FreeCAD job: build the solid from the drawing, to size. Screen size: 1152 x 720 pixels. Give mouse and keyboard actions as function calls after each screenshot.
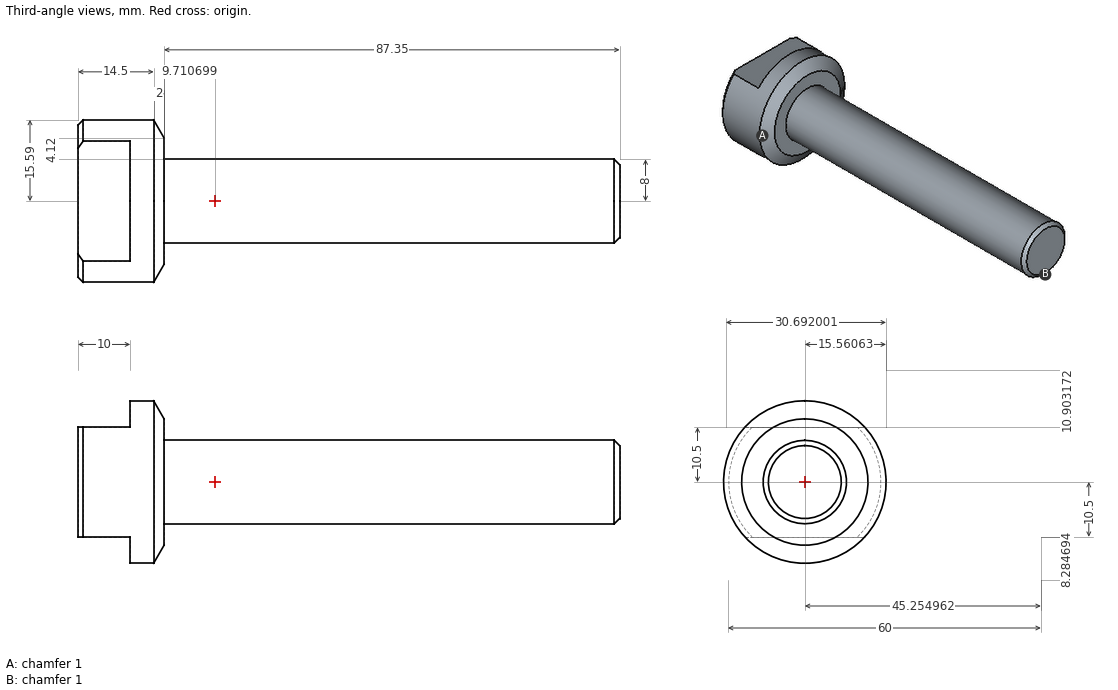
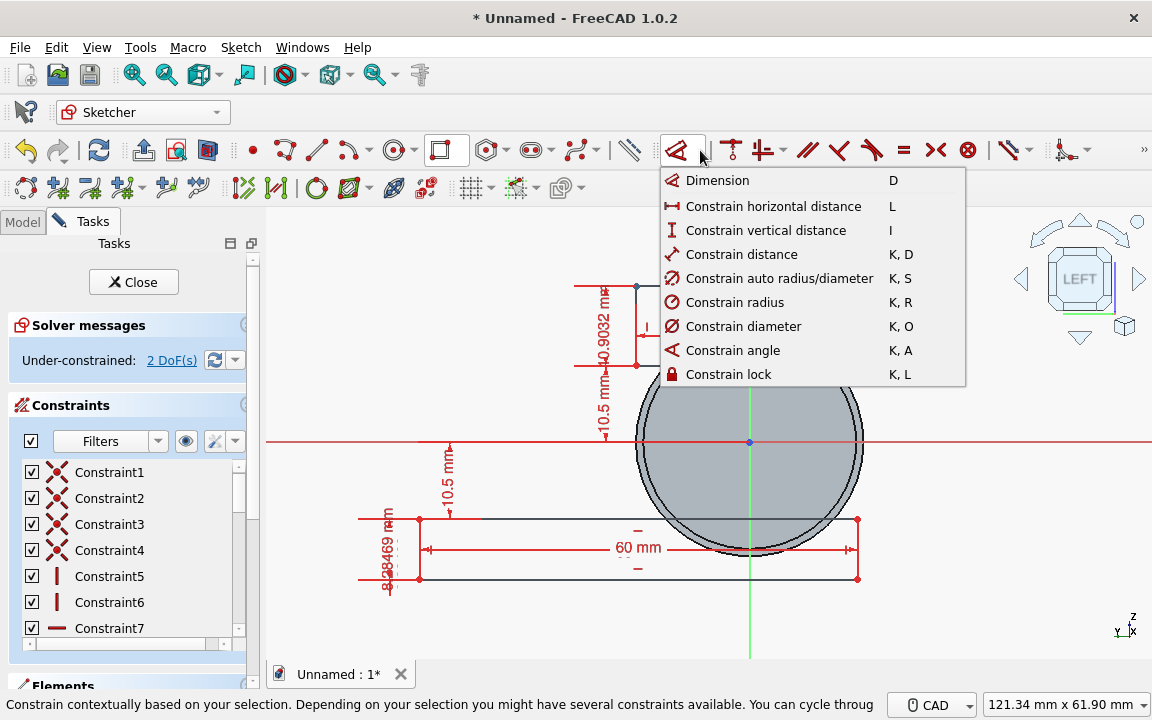
click(813, 206)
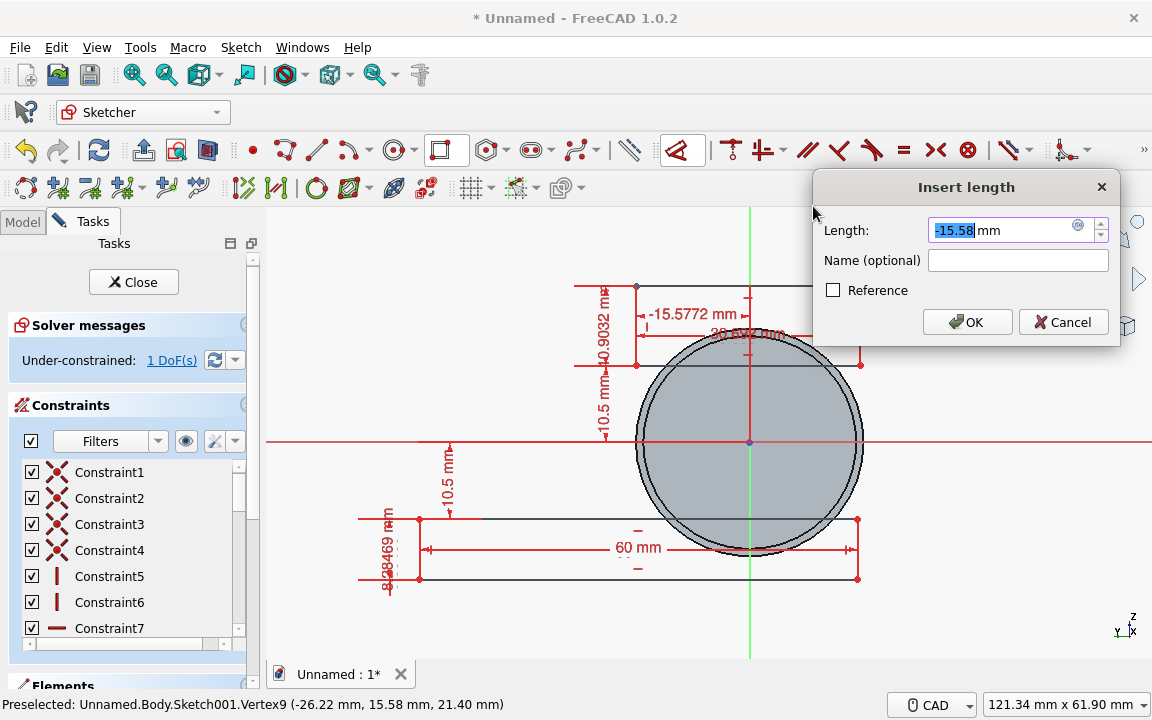
text(-15.56063)
key(Return)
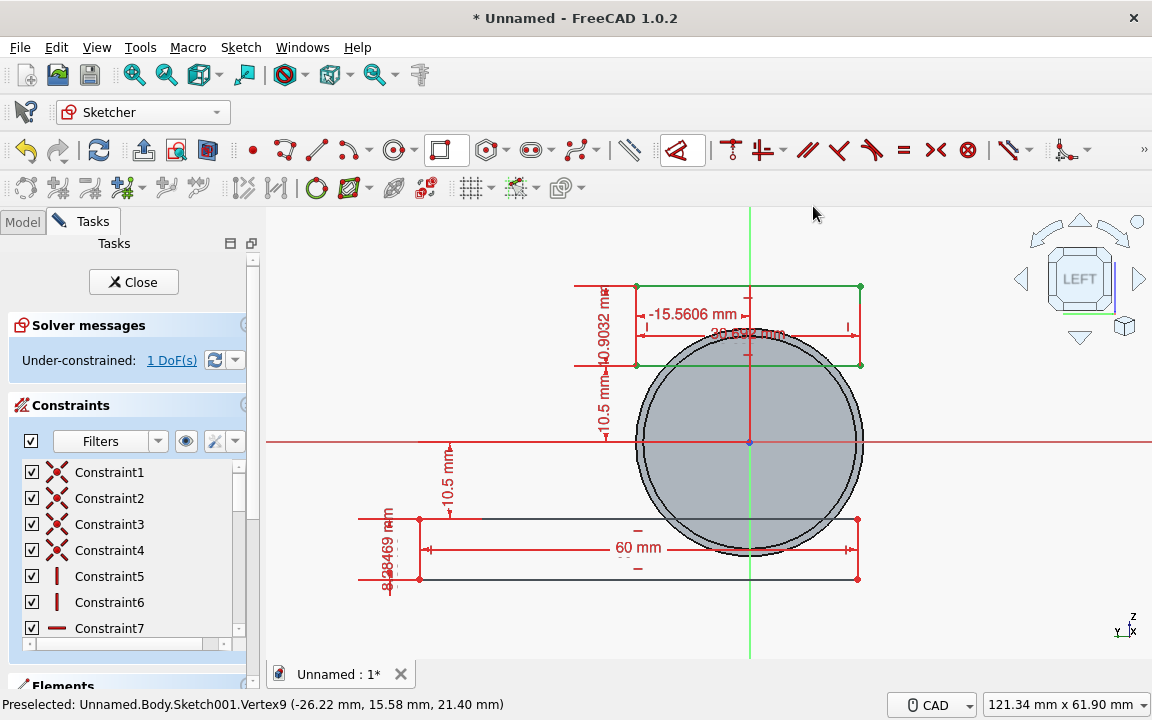
click(420, 519)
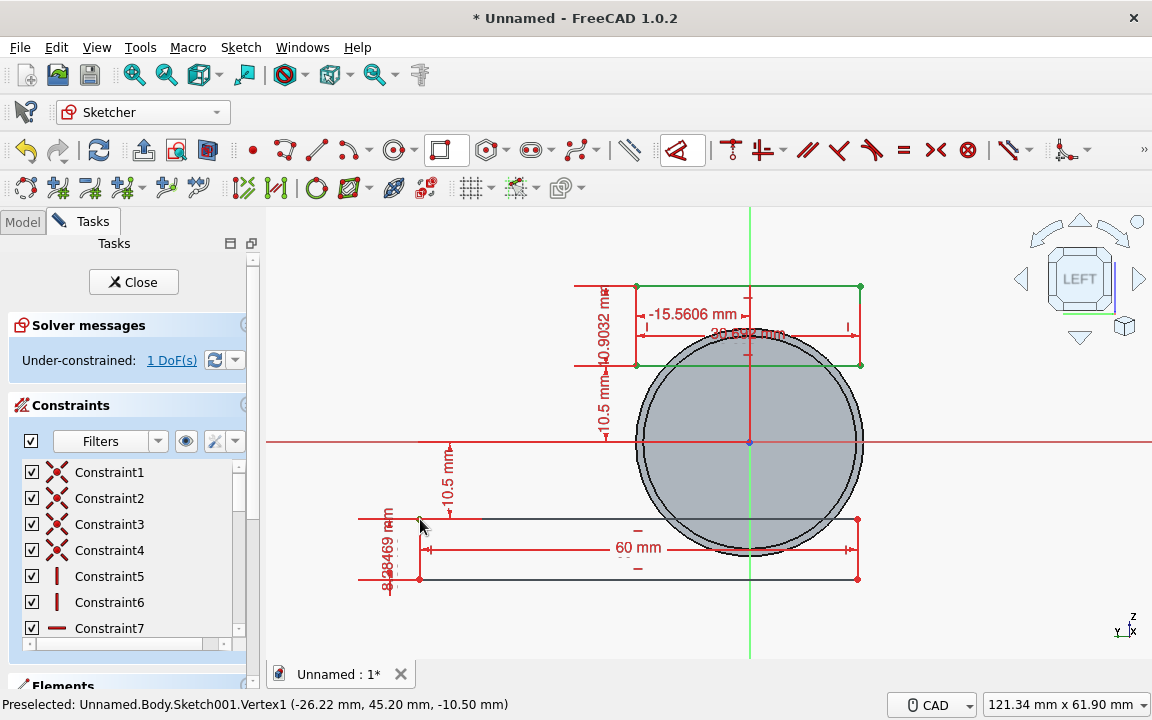
key(l)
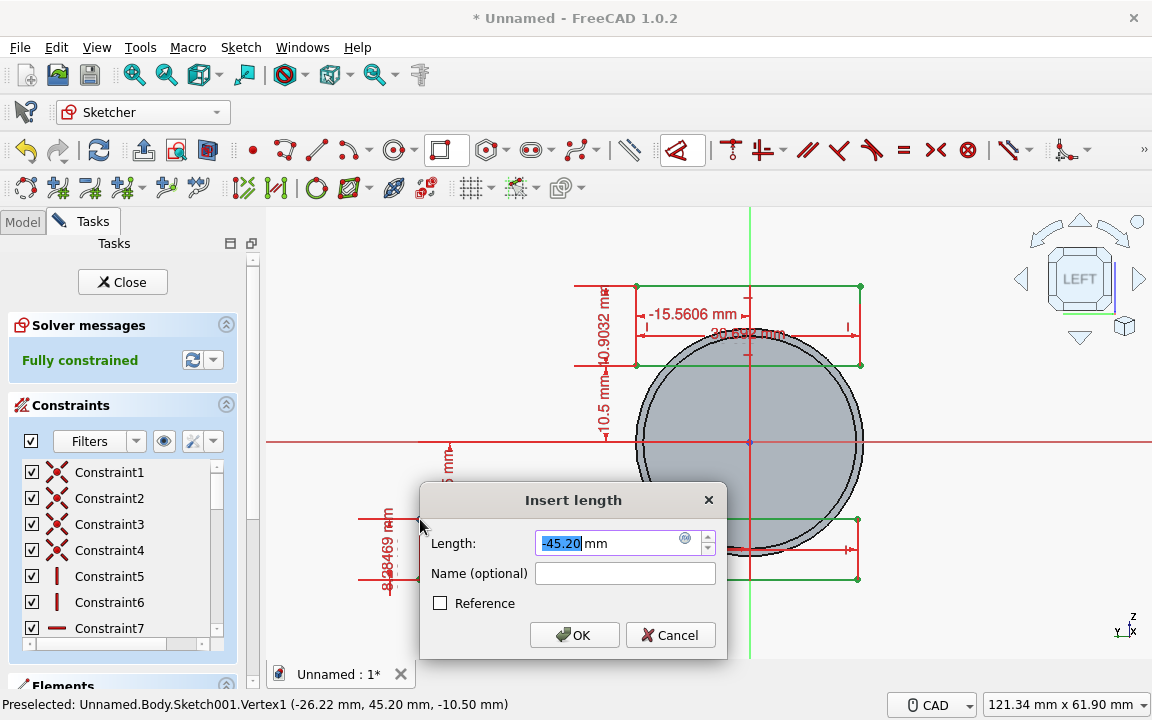
text(-45.254962)
key(Return)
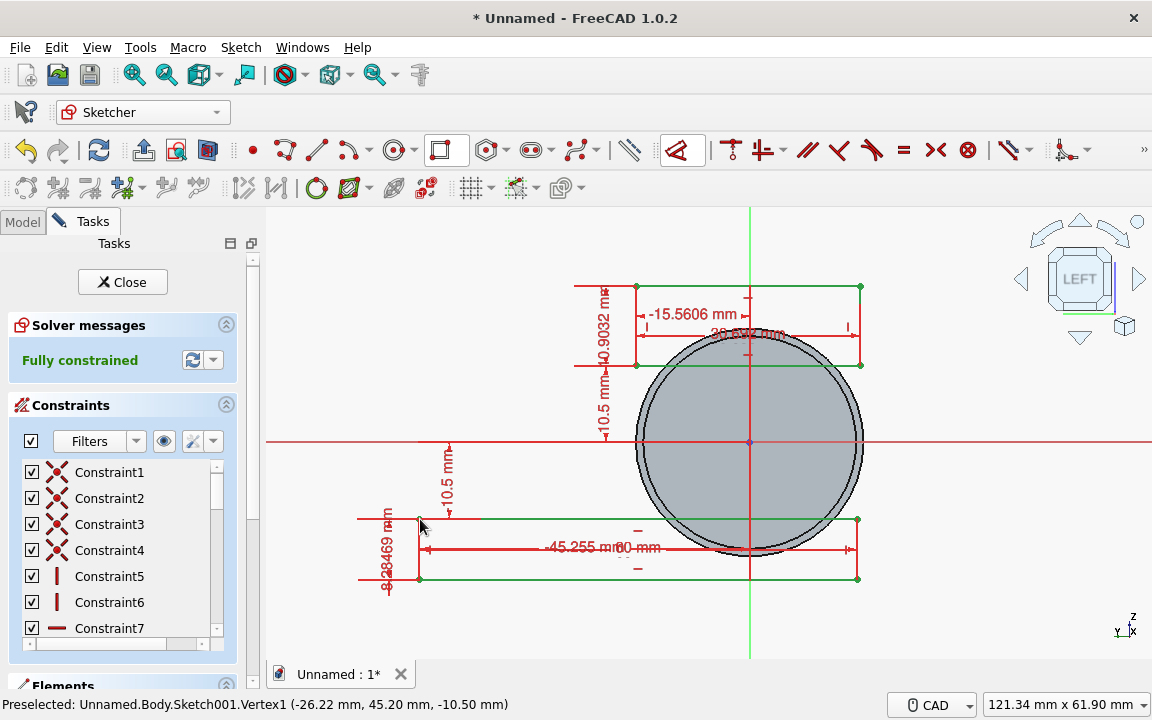
click(123, 282)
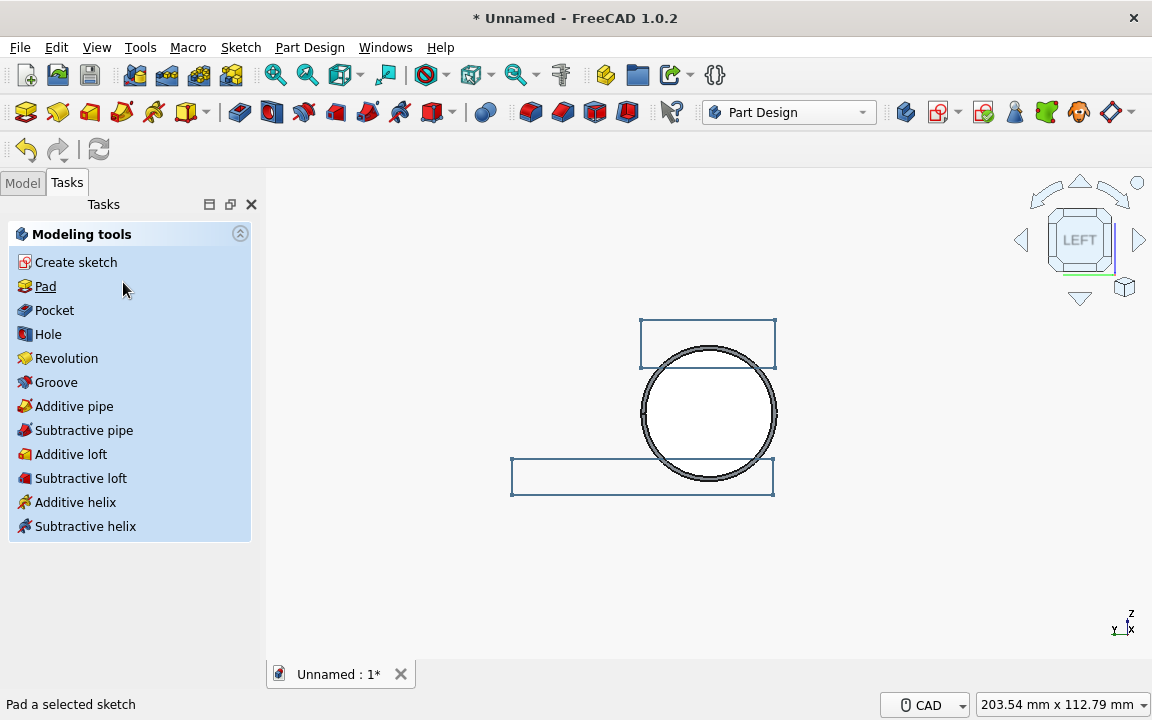
click(240, 112)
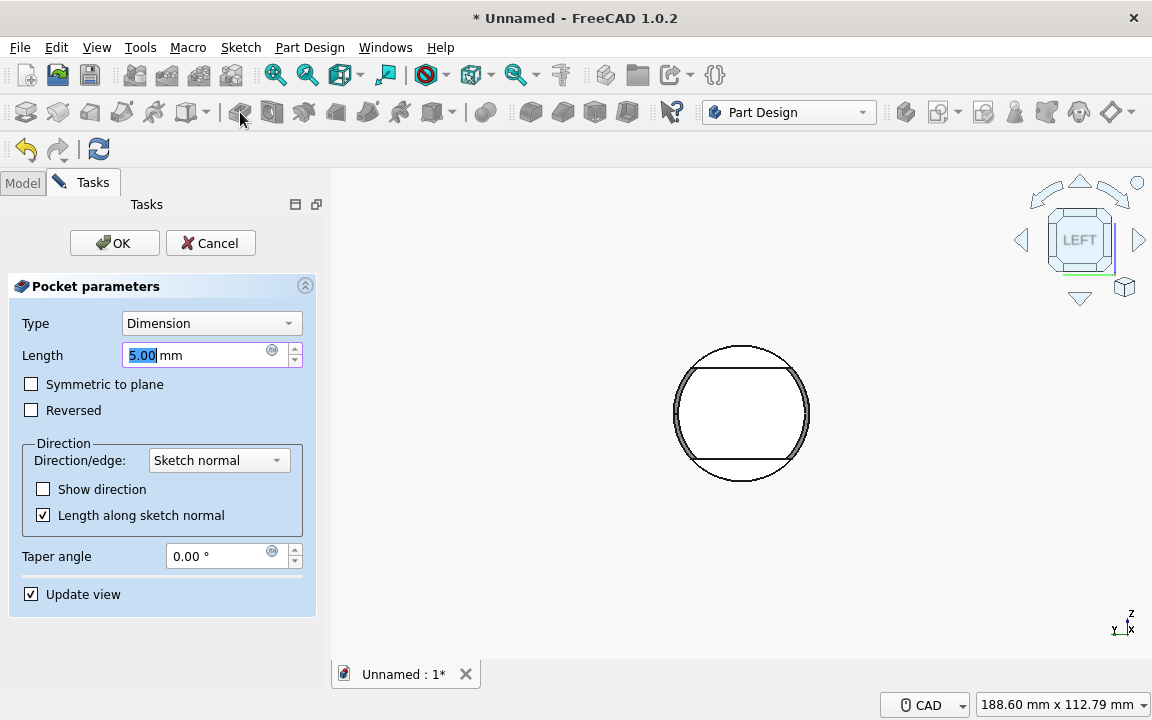
text(10)
key(Tab)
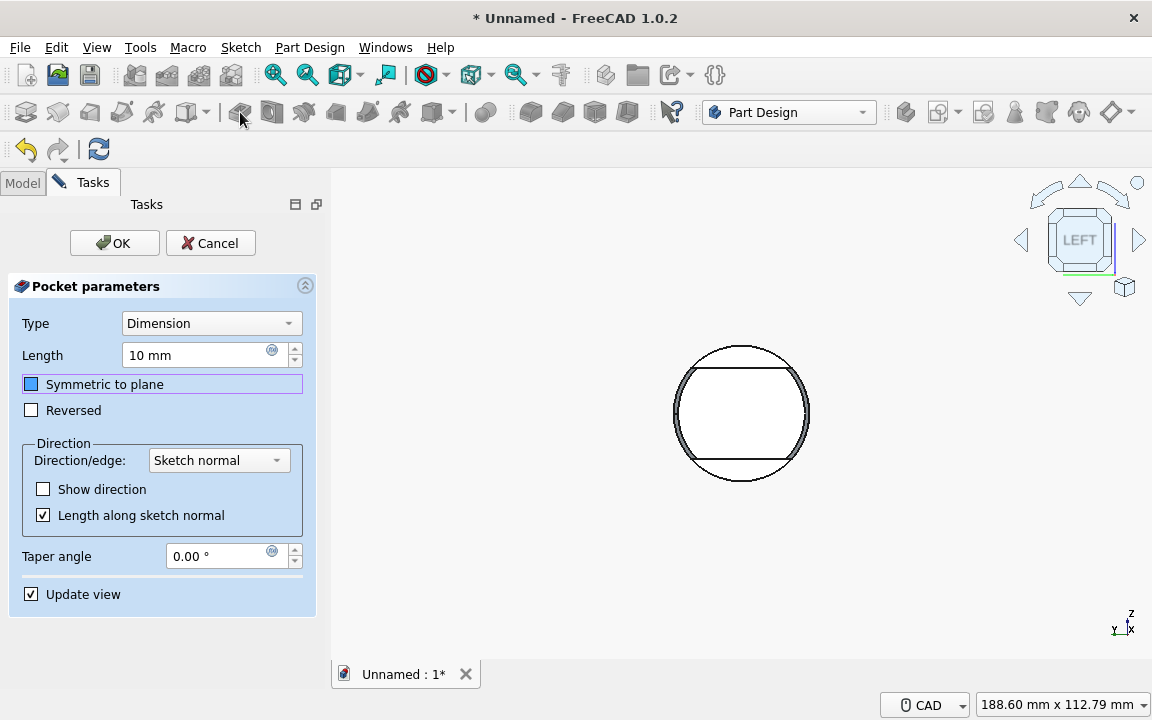
click(115, 243)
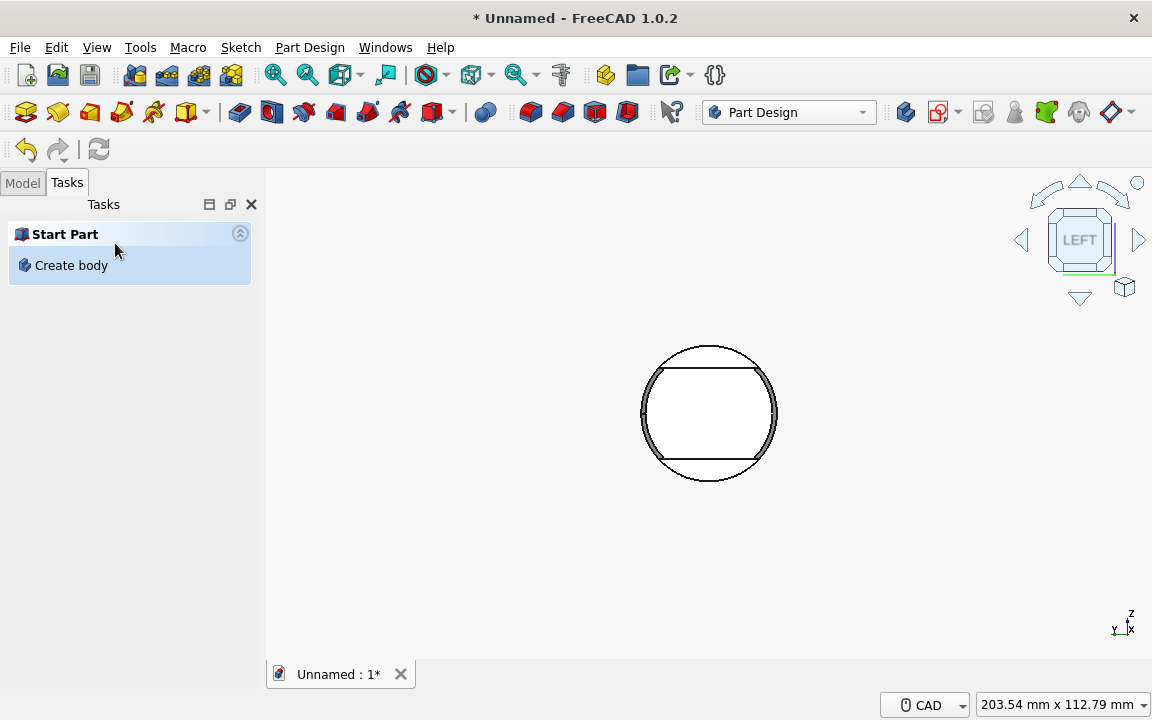
key(0)